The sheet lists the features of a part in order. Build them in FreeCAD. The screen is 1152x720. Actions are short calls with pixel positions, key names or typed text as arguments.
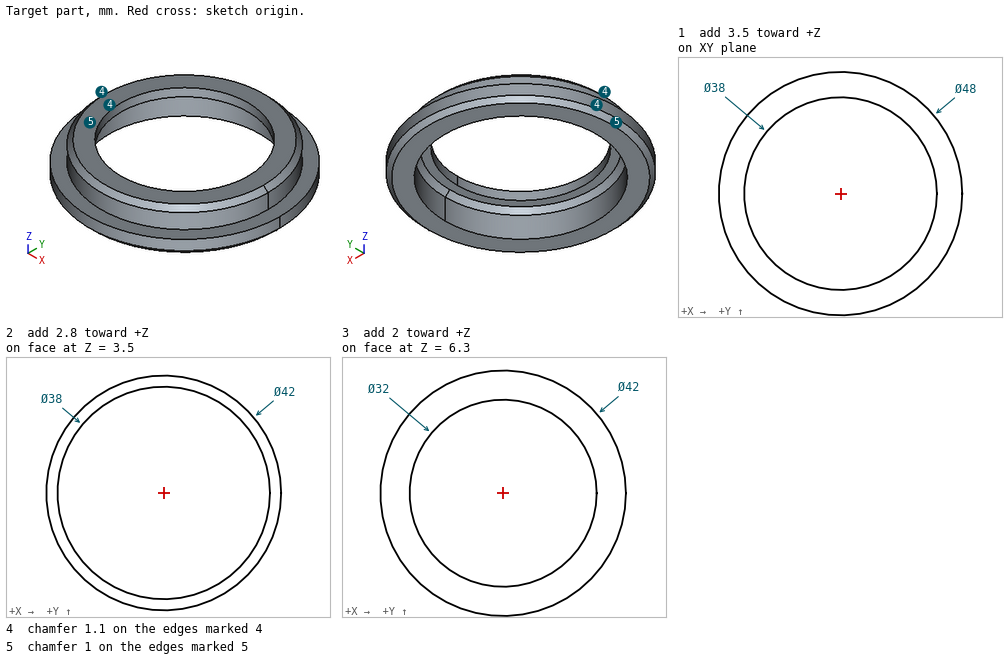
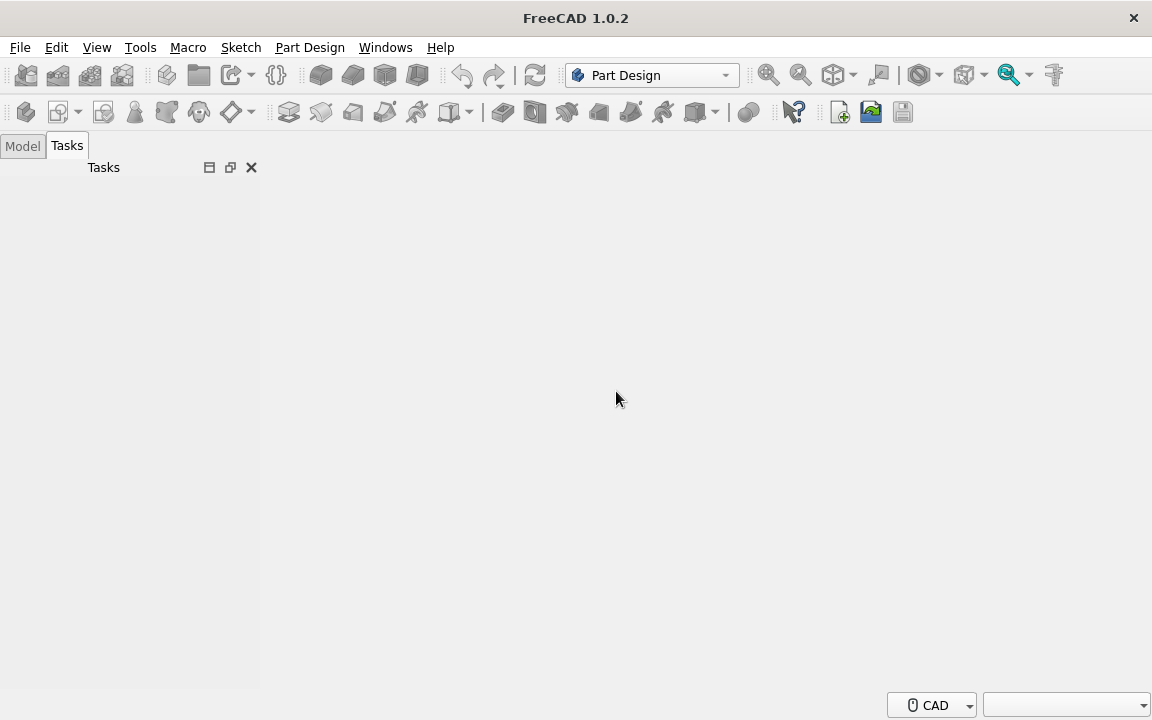
click(840, 112)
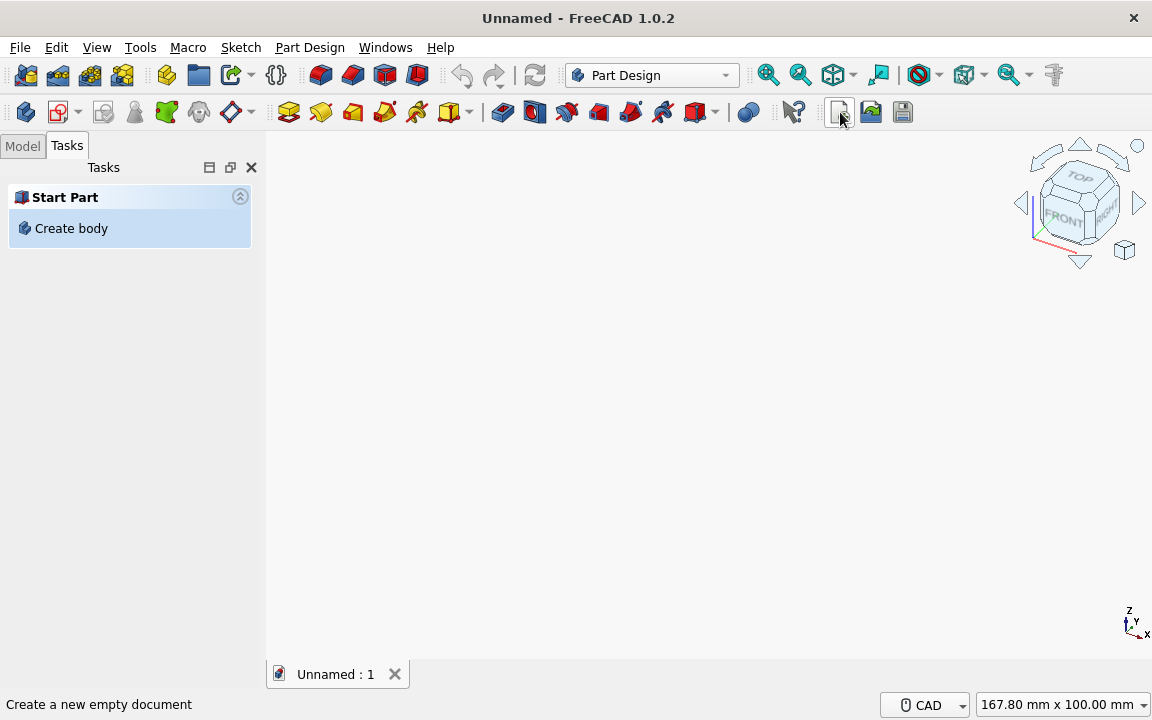
click(58, 112)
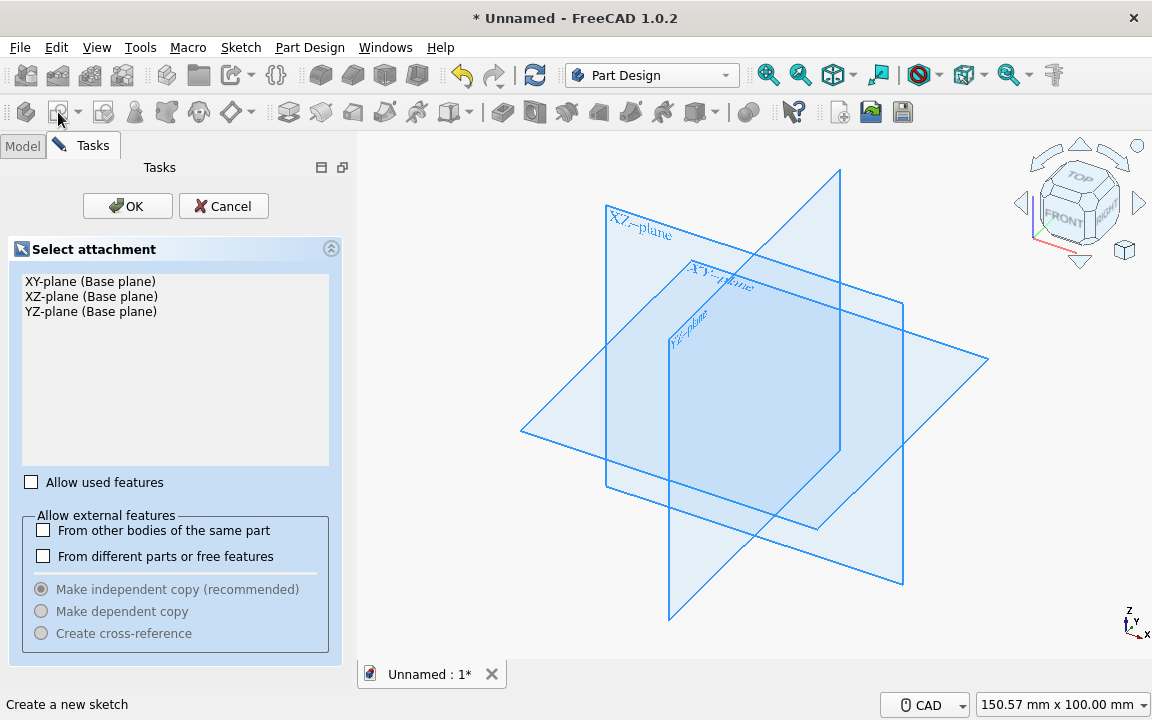
click(82, 282)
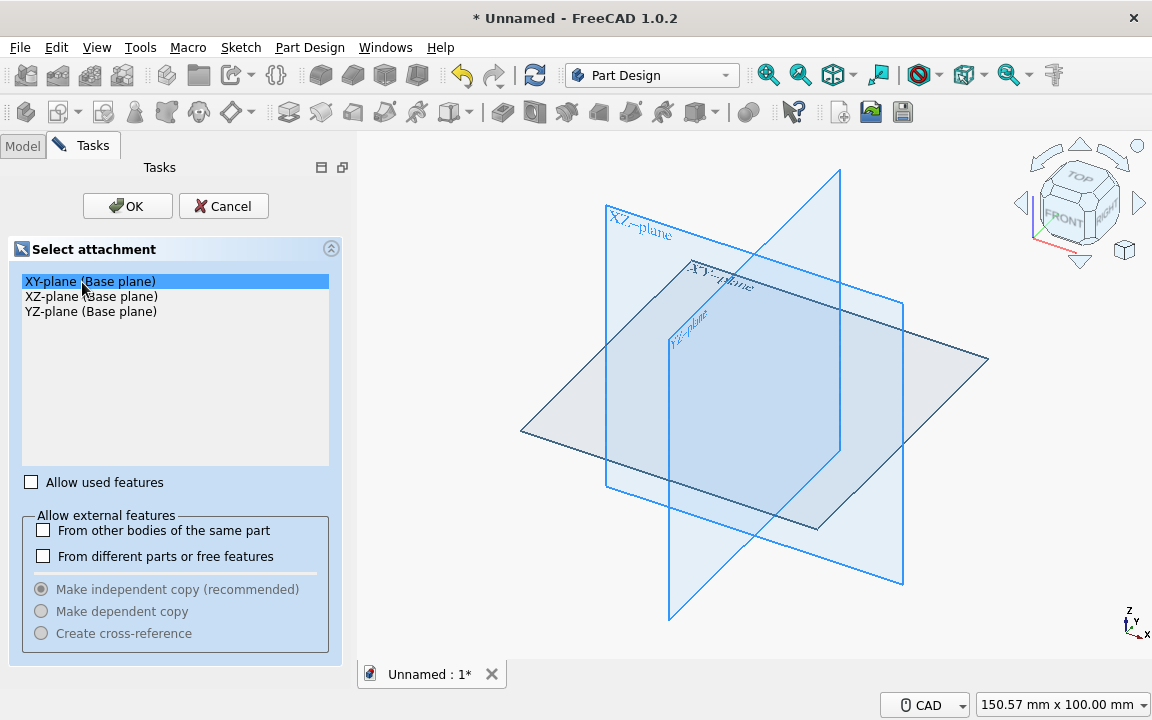
click(128, 206)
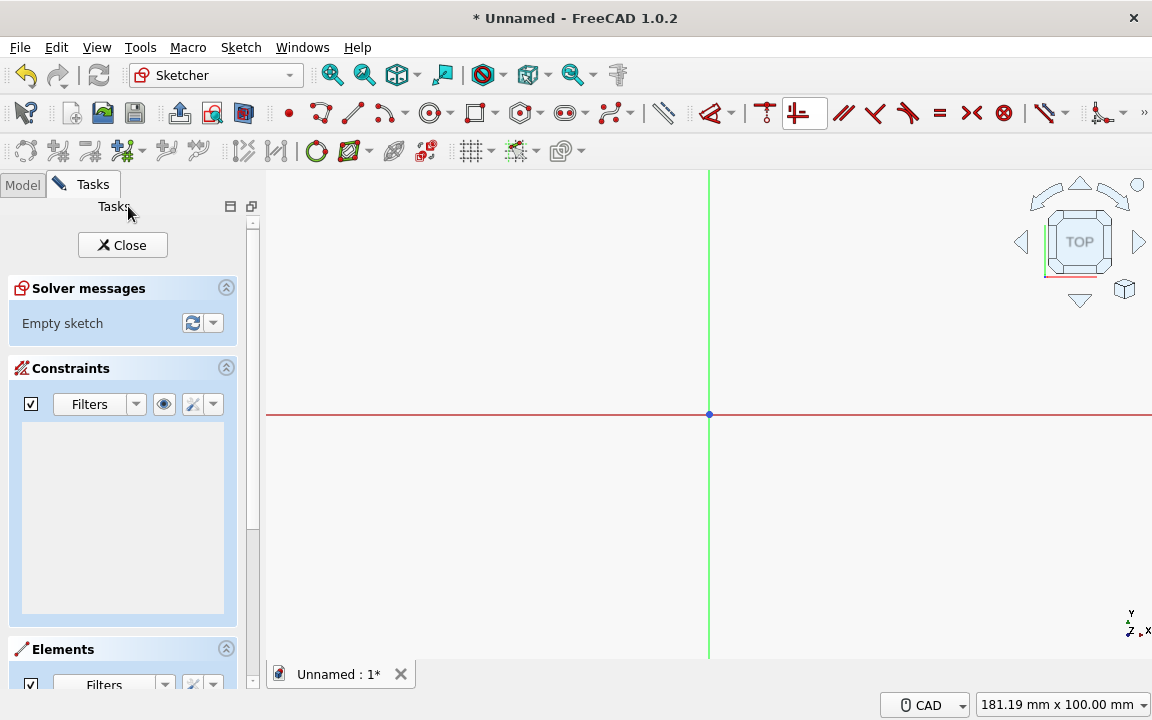
click(430, 114)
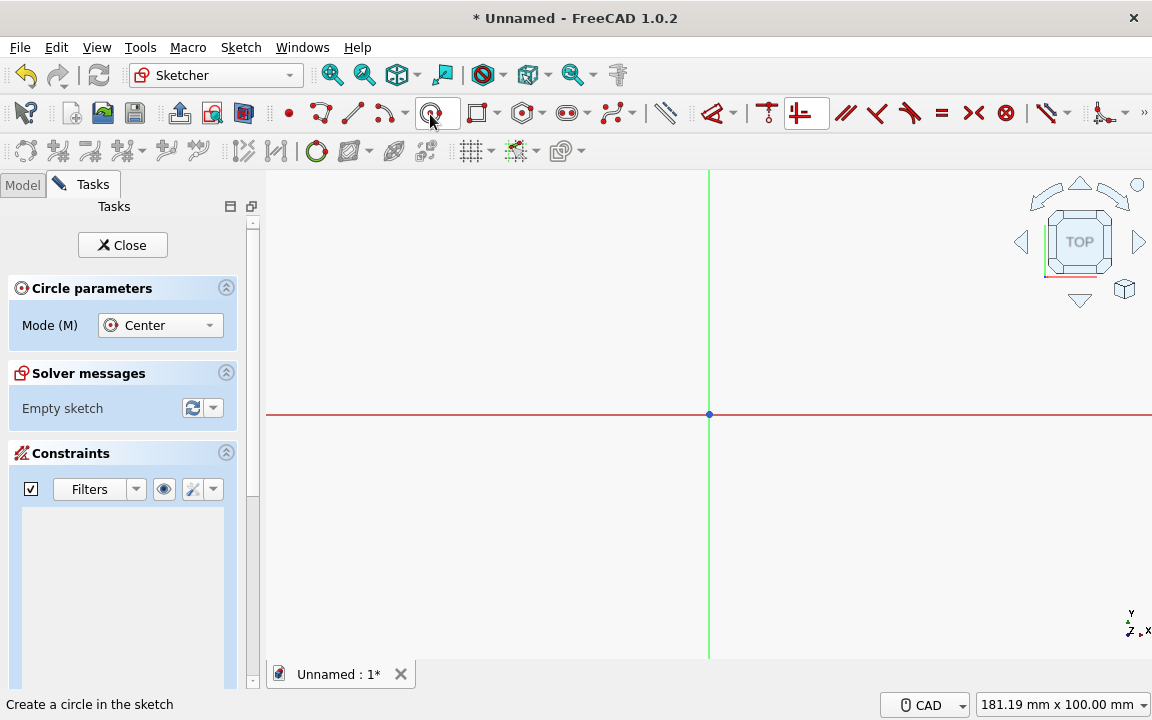
click(709, 414)
move(792, 332)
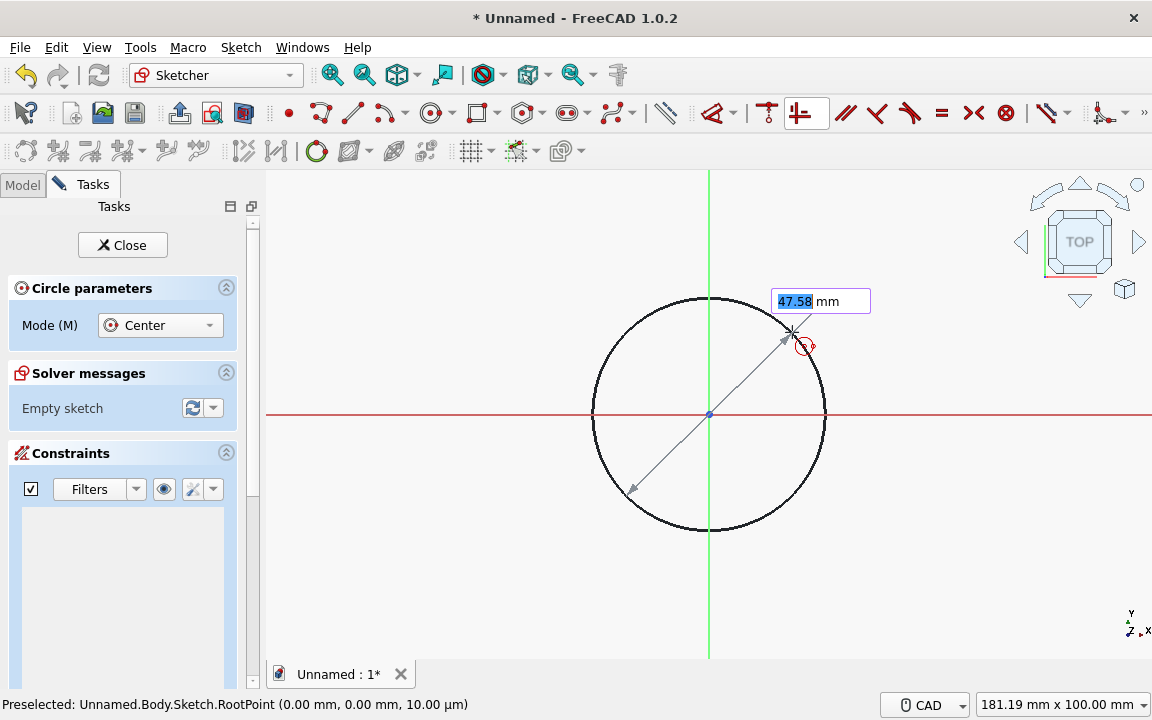
text(48)
key(Return)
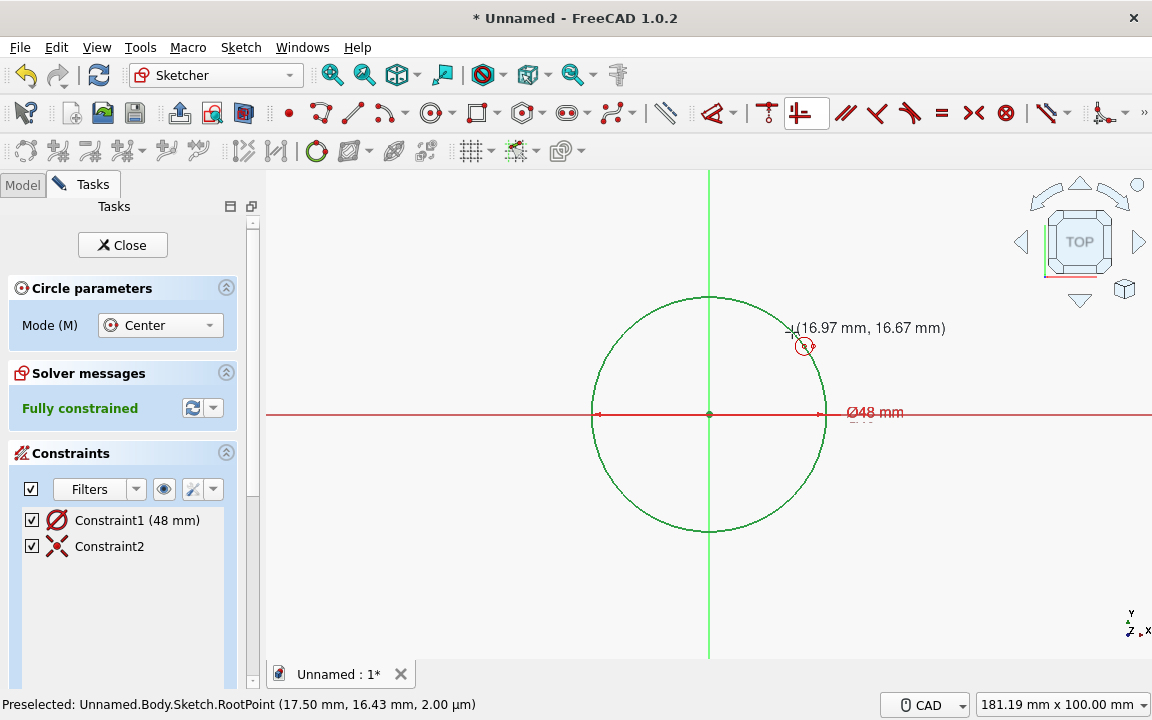
click(709, 414)
move(775, 349)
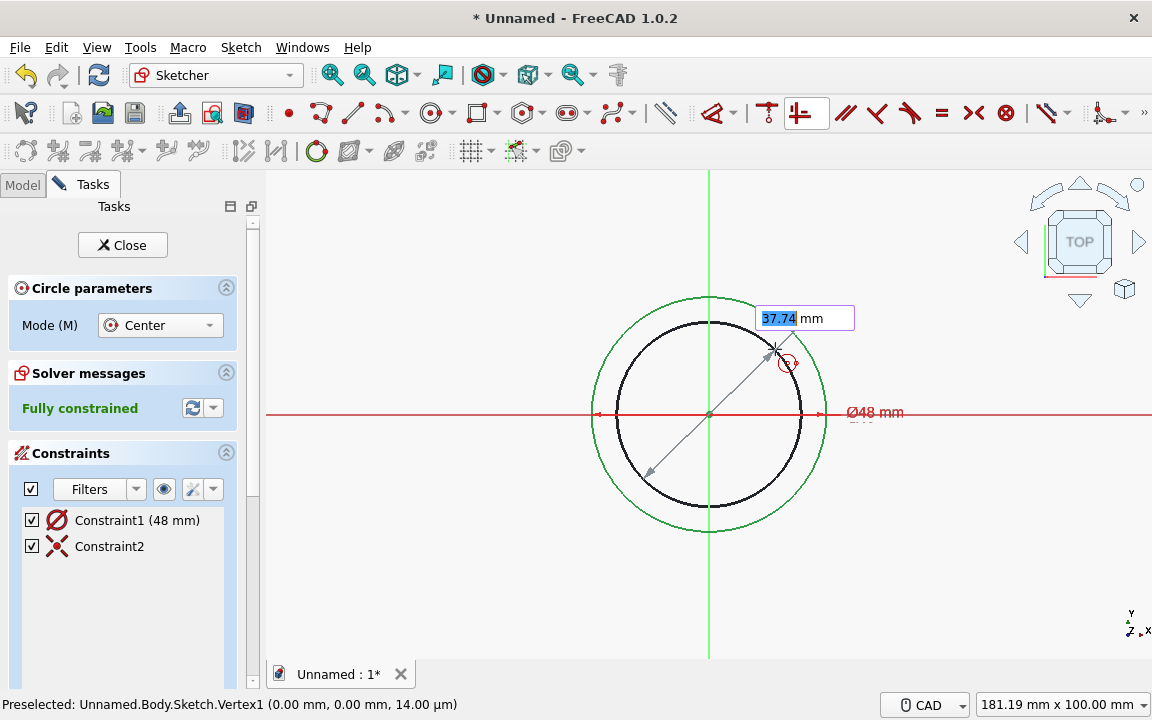
text(38)
key(Return)
key(Escape)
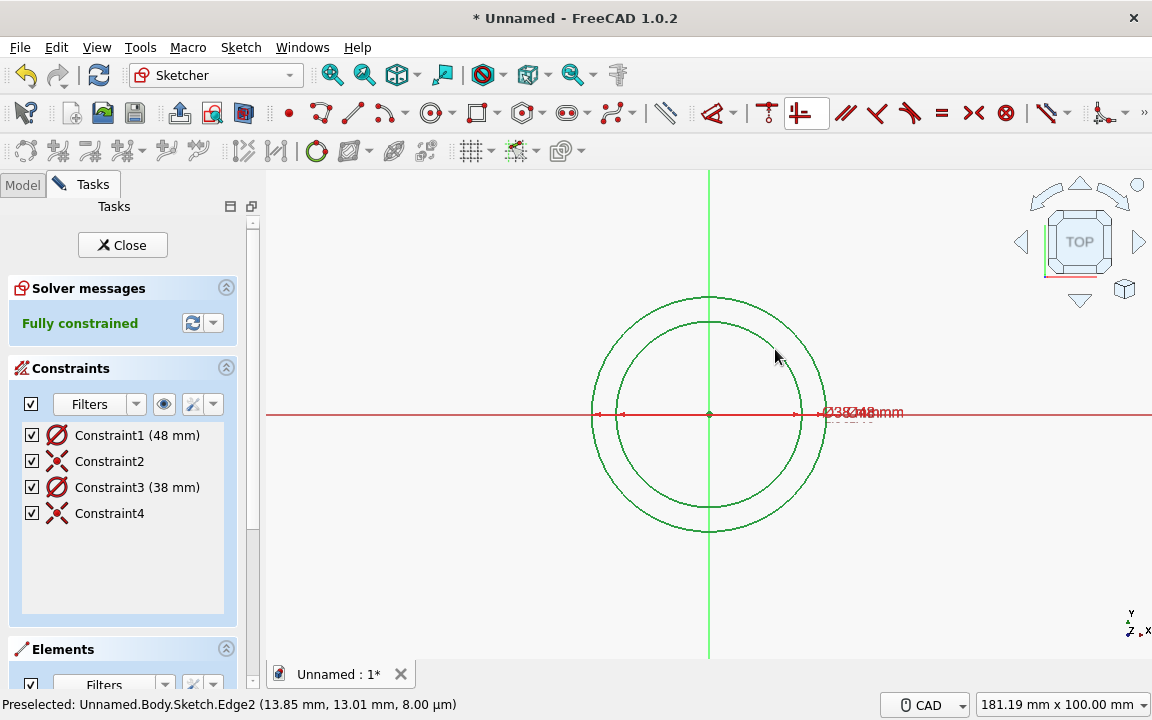
click(123, 245)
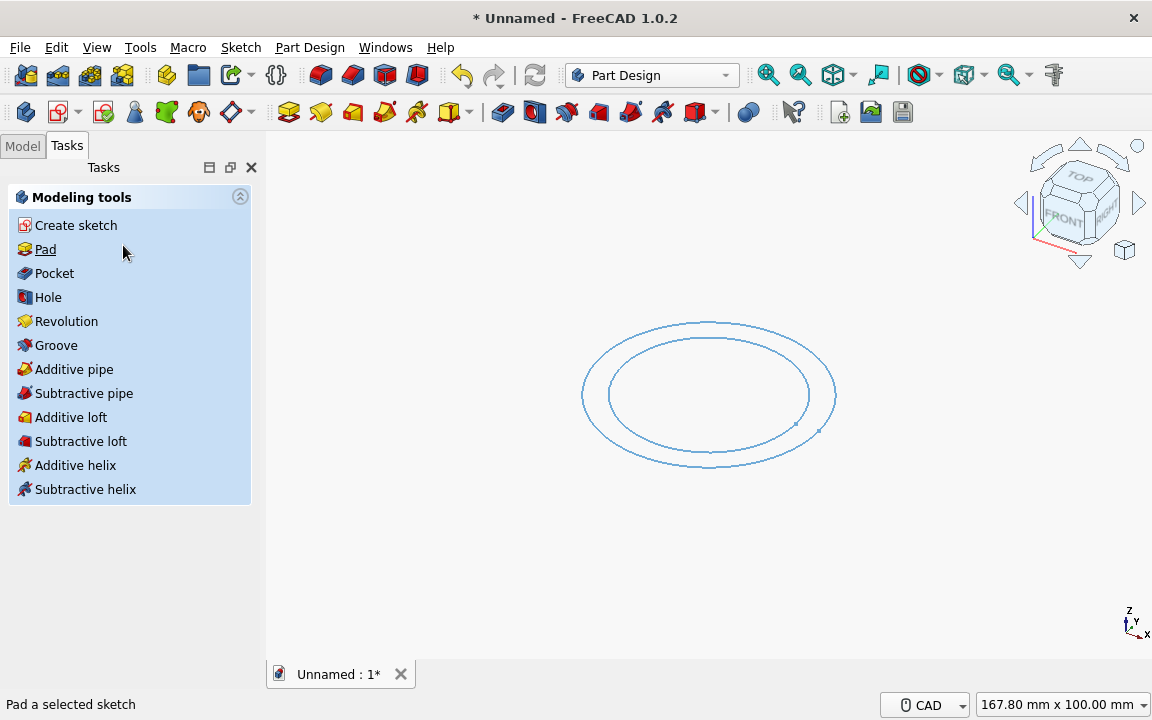
click(290, 112)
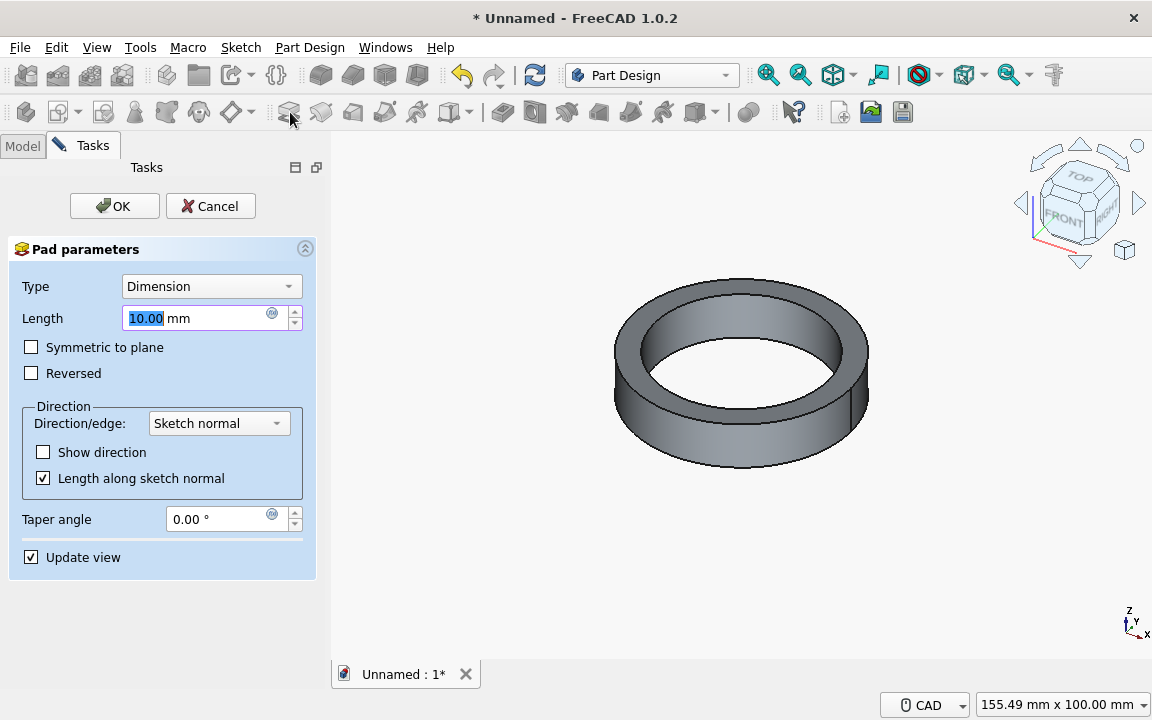
text(3.5)
key(Tab)